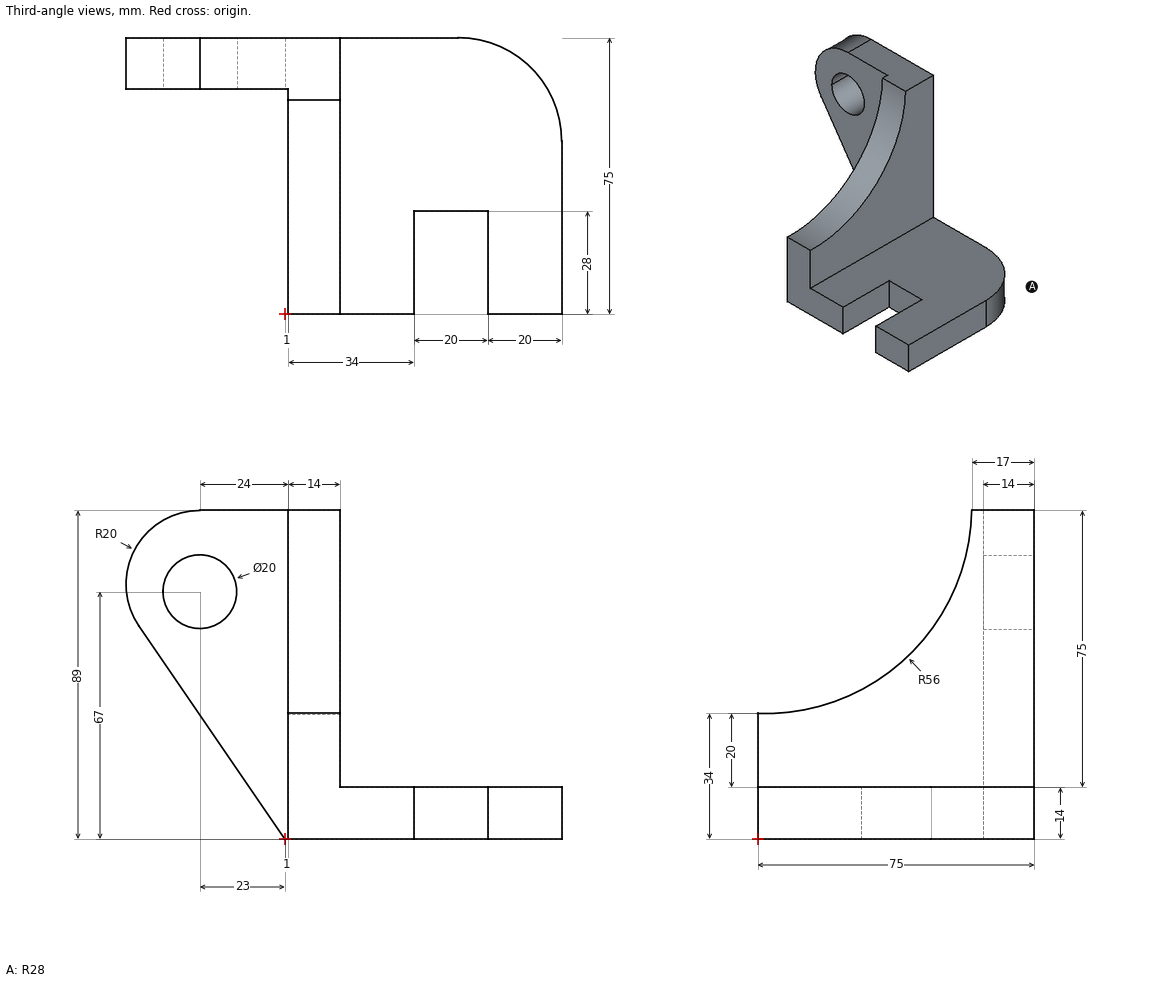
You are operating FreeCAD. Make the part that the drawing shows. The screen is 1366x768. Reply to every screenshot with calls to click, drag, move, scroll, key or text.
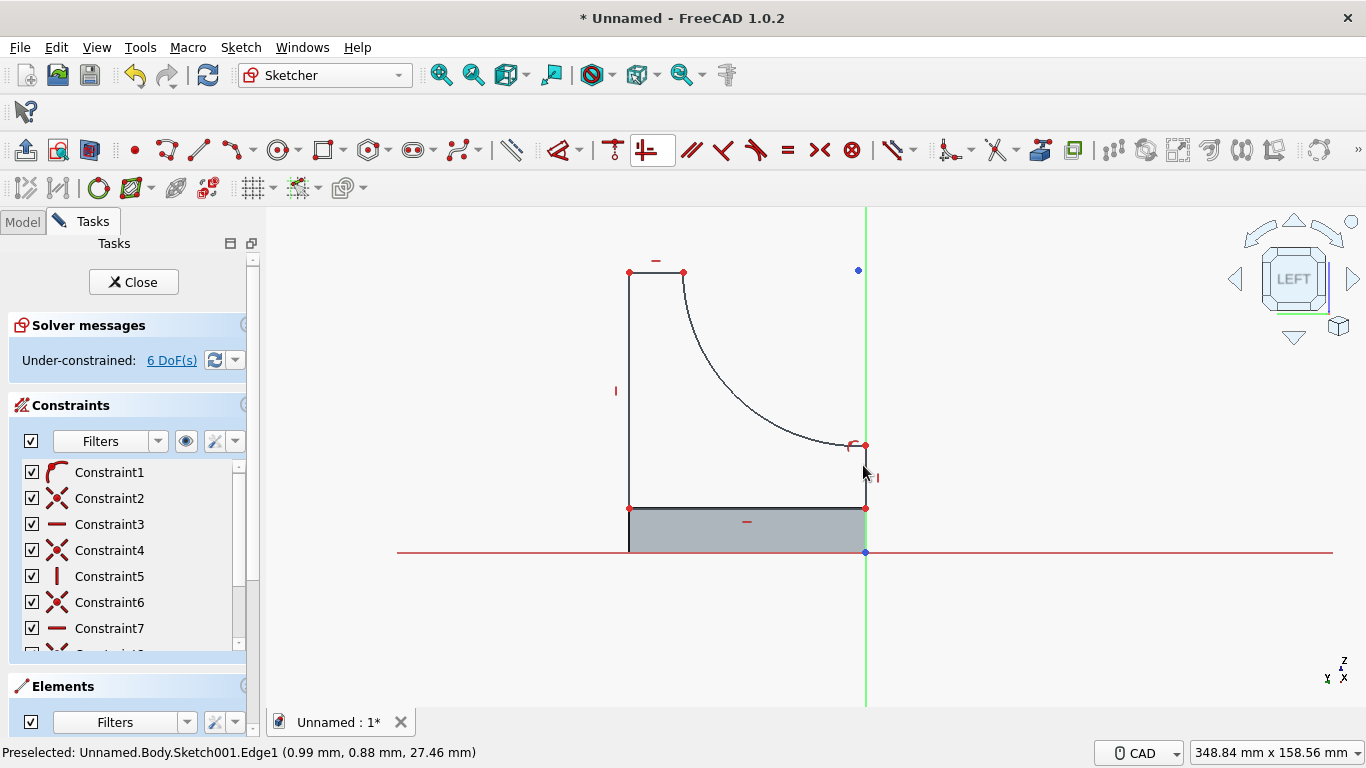
click(558, 150)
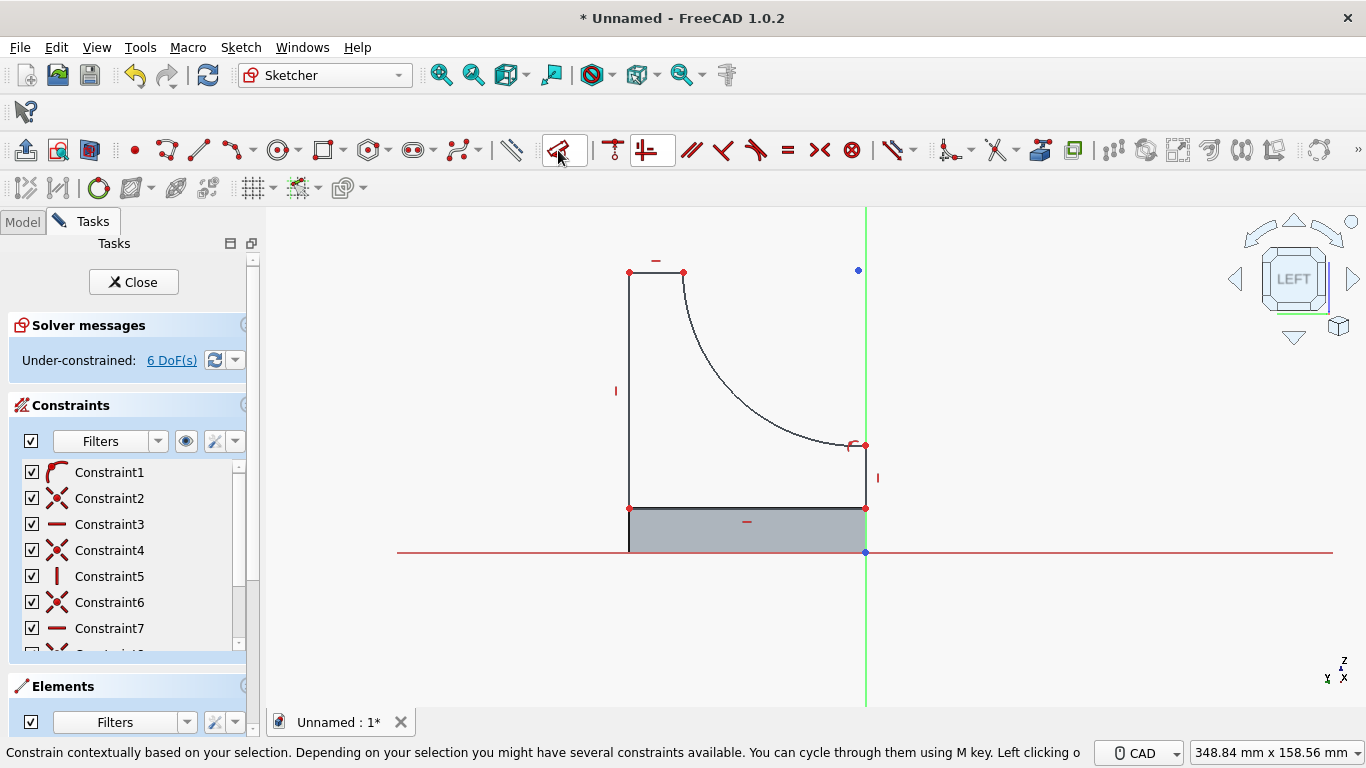
click(704, 354)
click(676, 369)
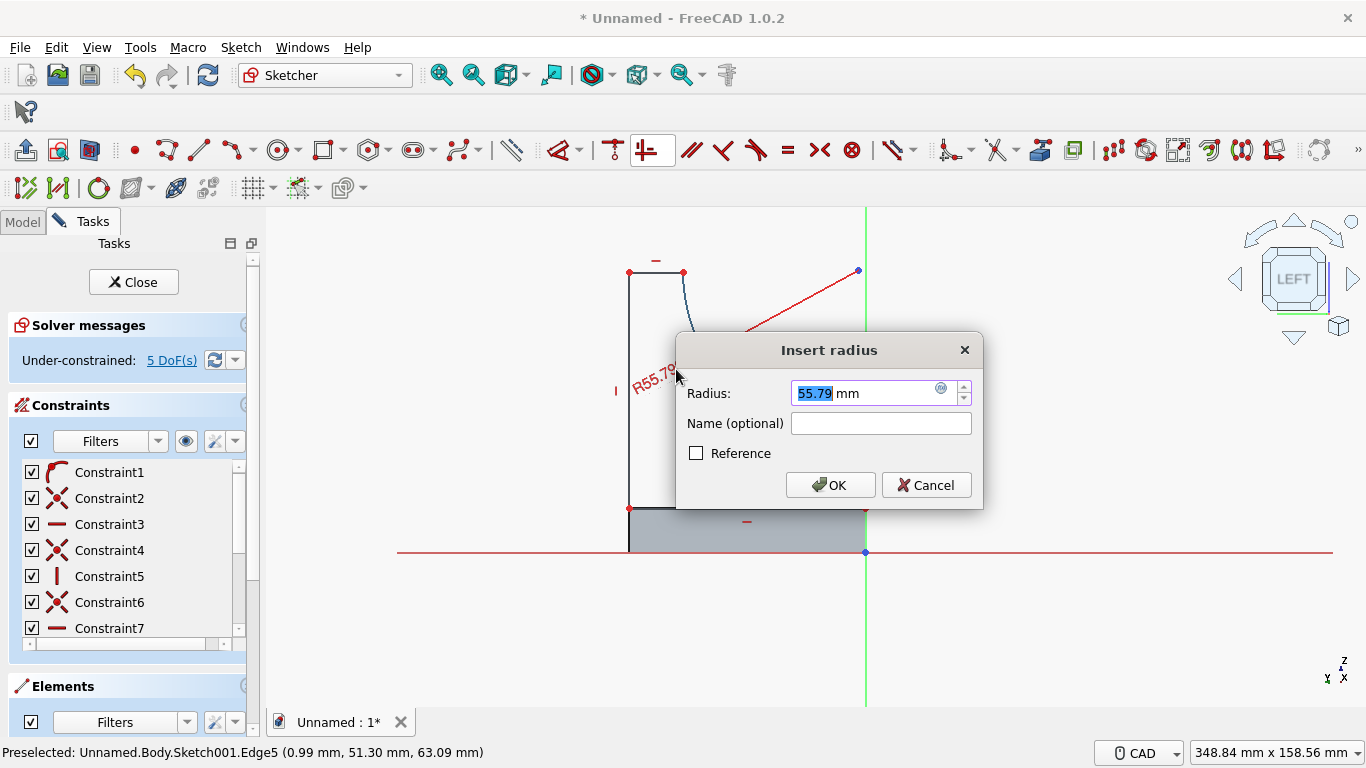
text(56)
key(Return)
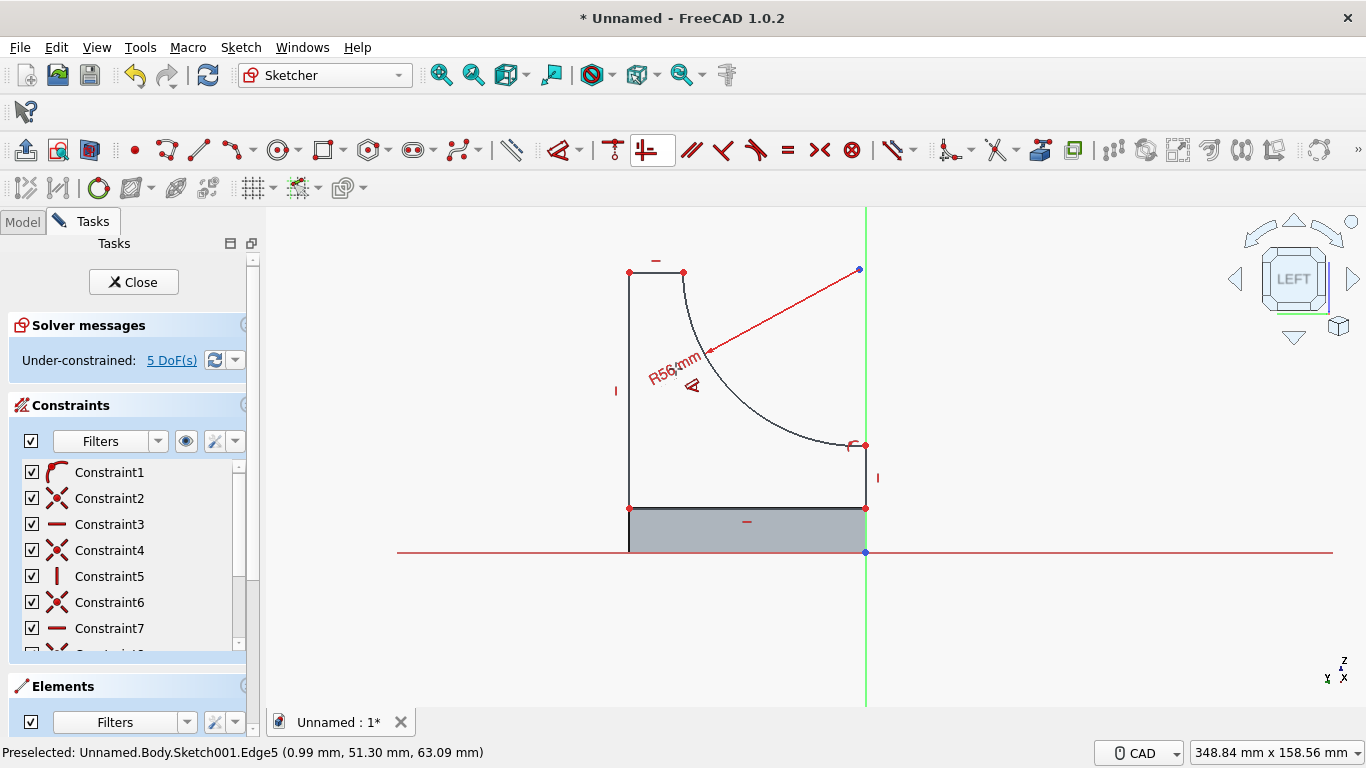
click(866, 465)
click(900, 477)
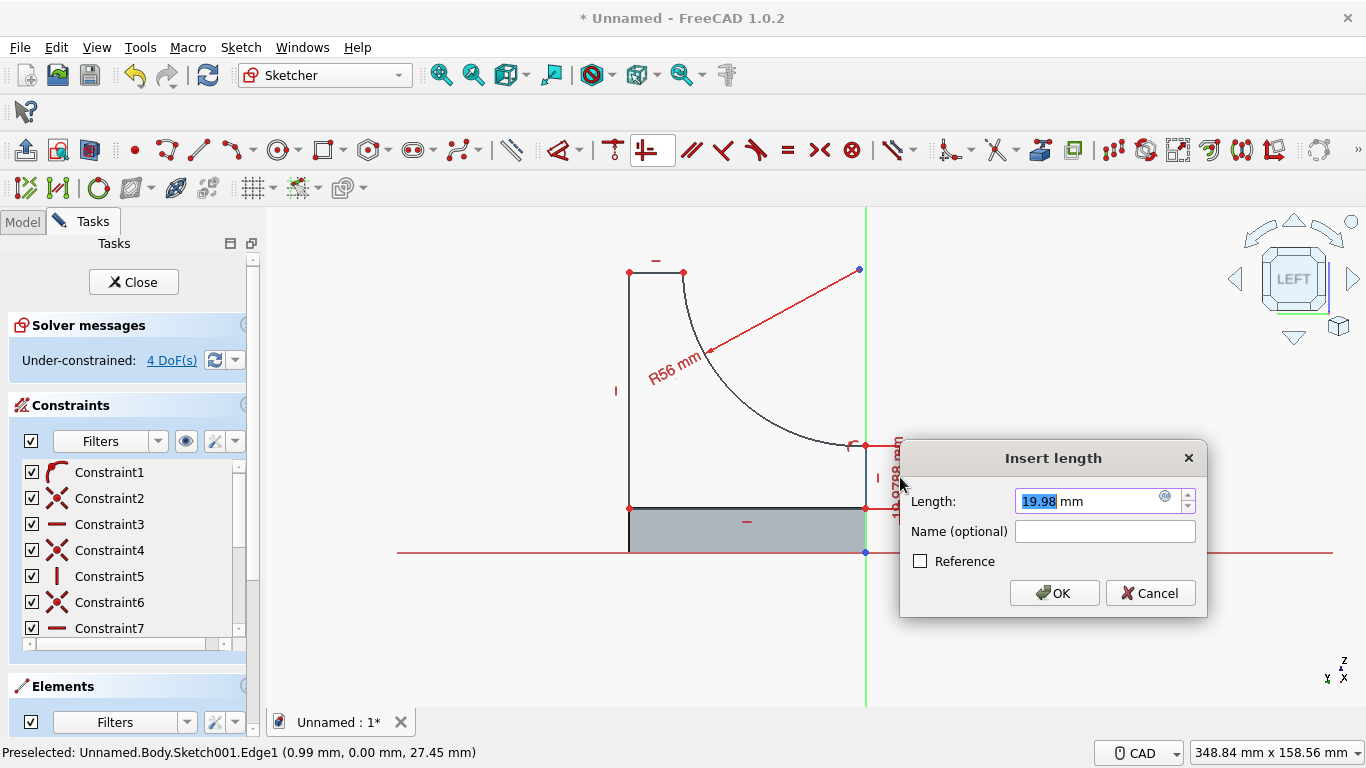
text(20)
key(Return)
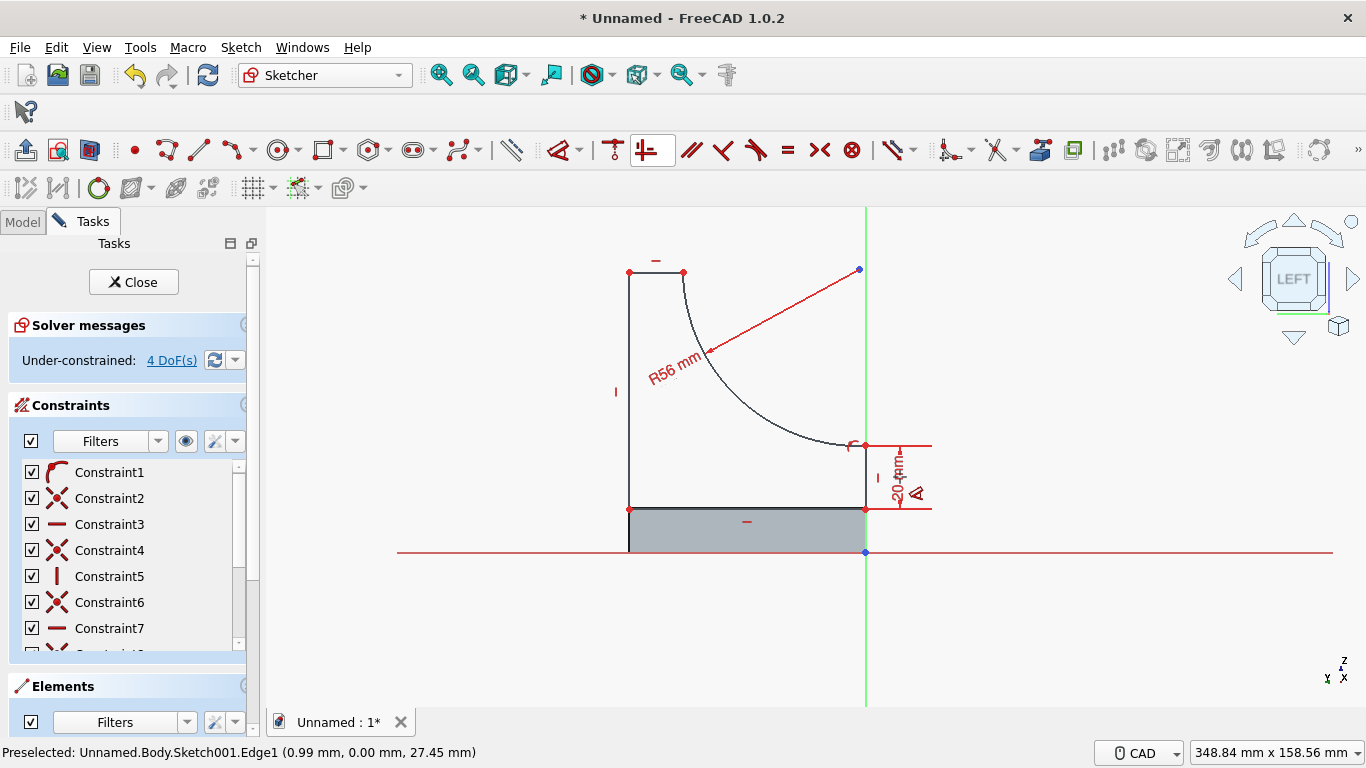
click(795, 509)
click(747, 475)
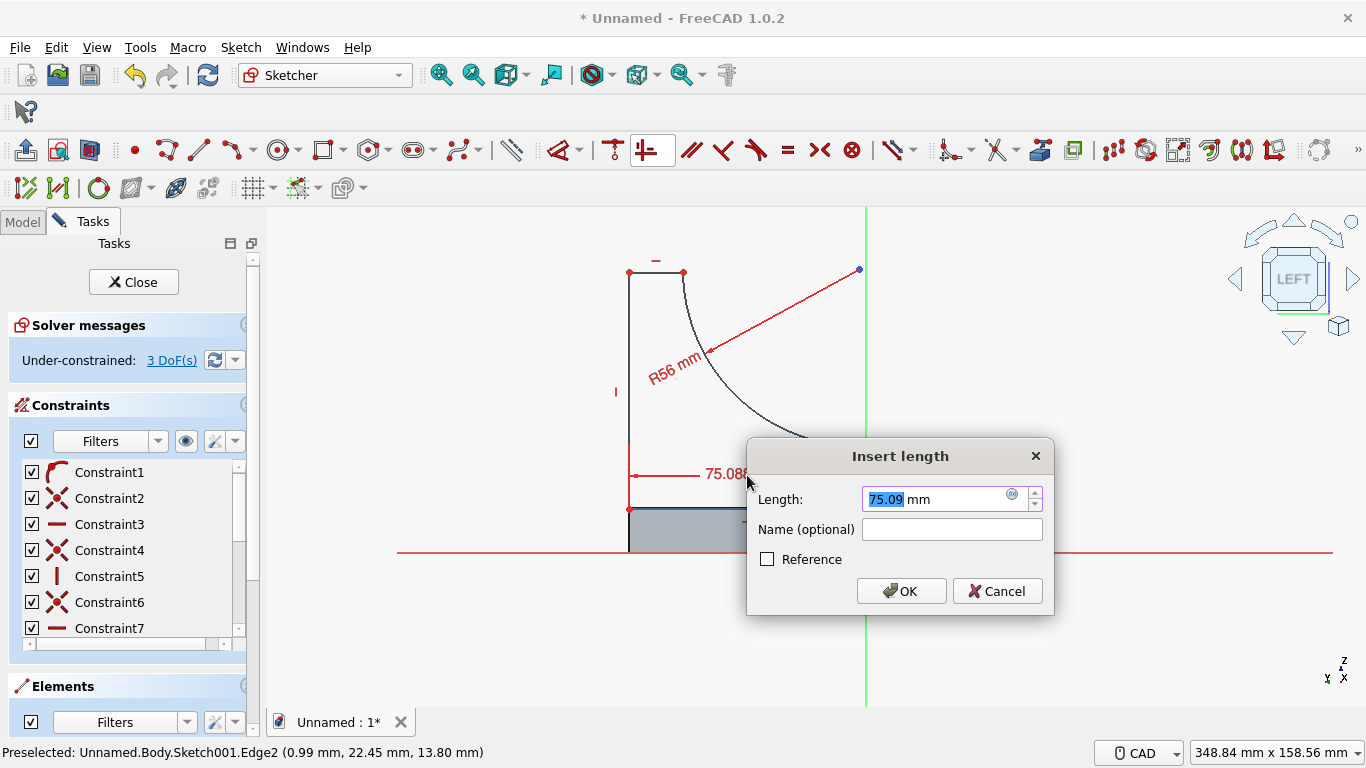
text(75)
key(Return)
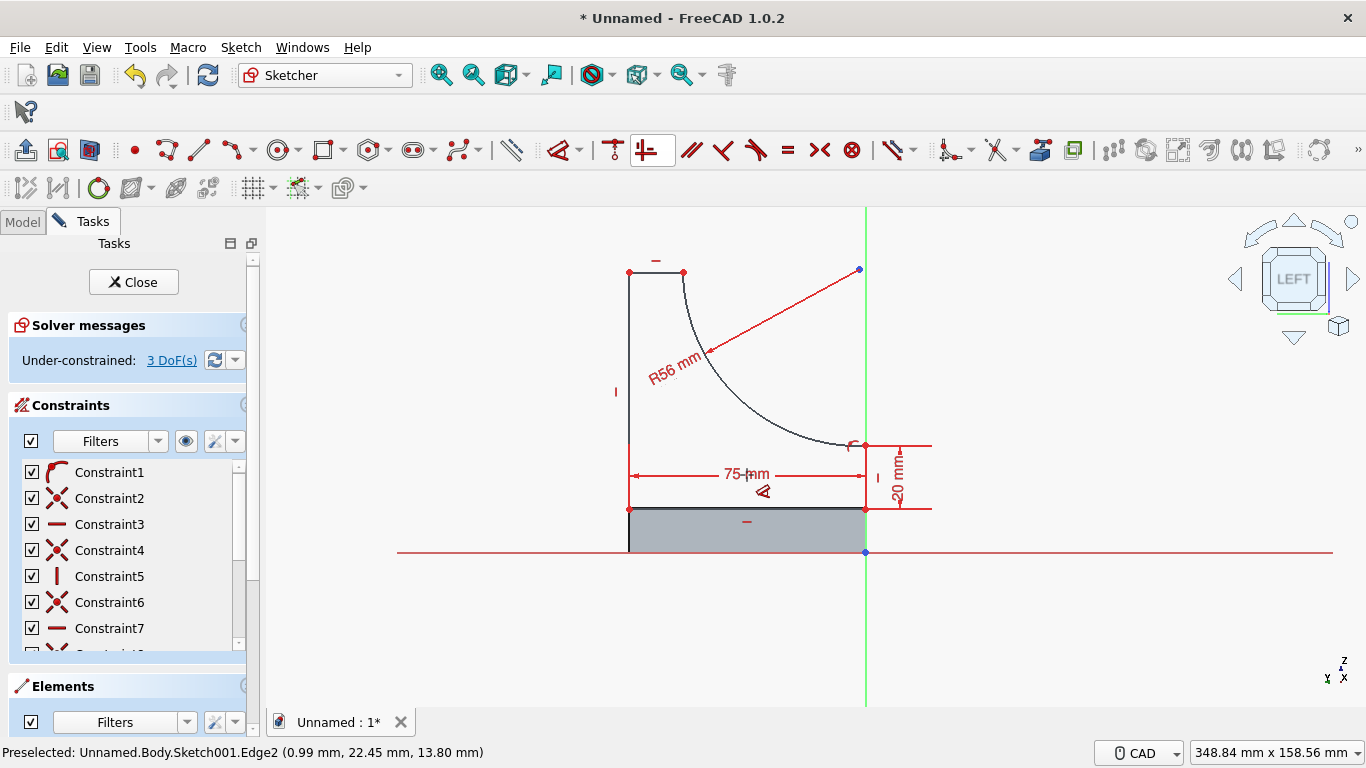
click(629, 438)
click(595, 391)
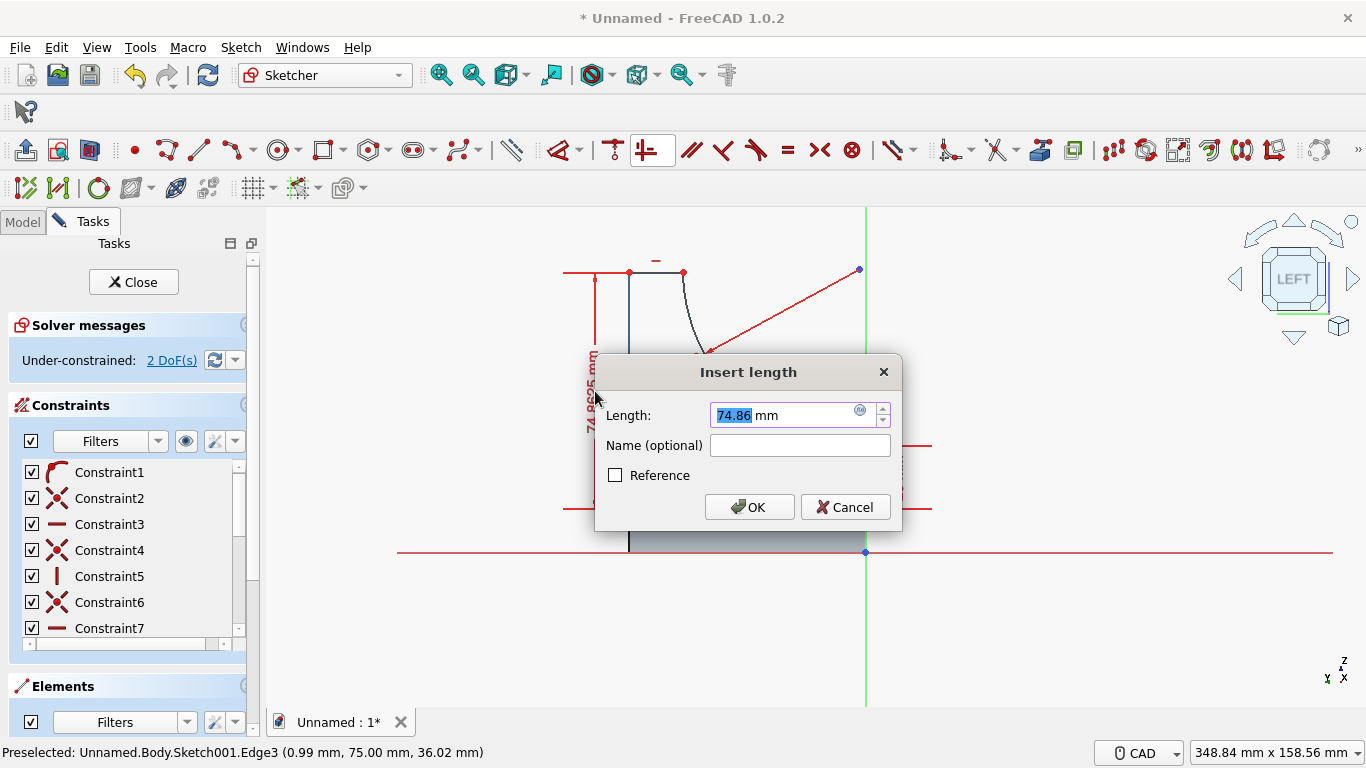
text(75)
key(Return)